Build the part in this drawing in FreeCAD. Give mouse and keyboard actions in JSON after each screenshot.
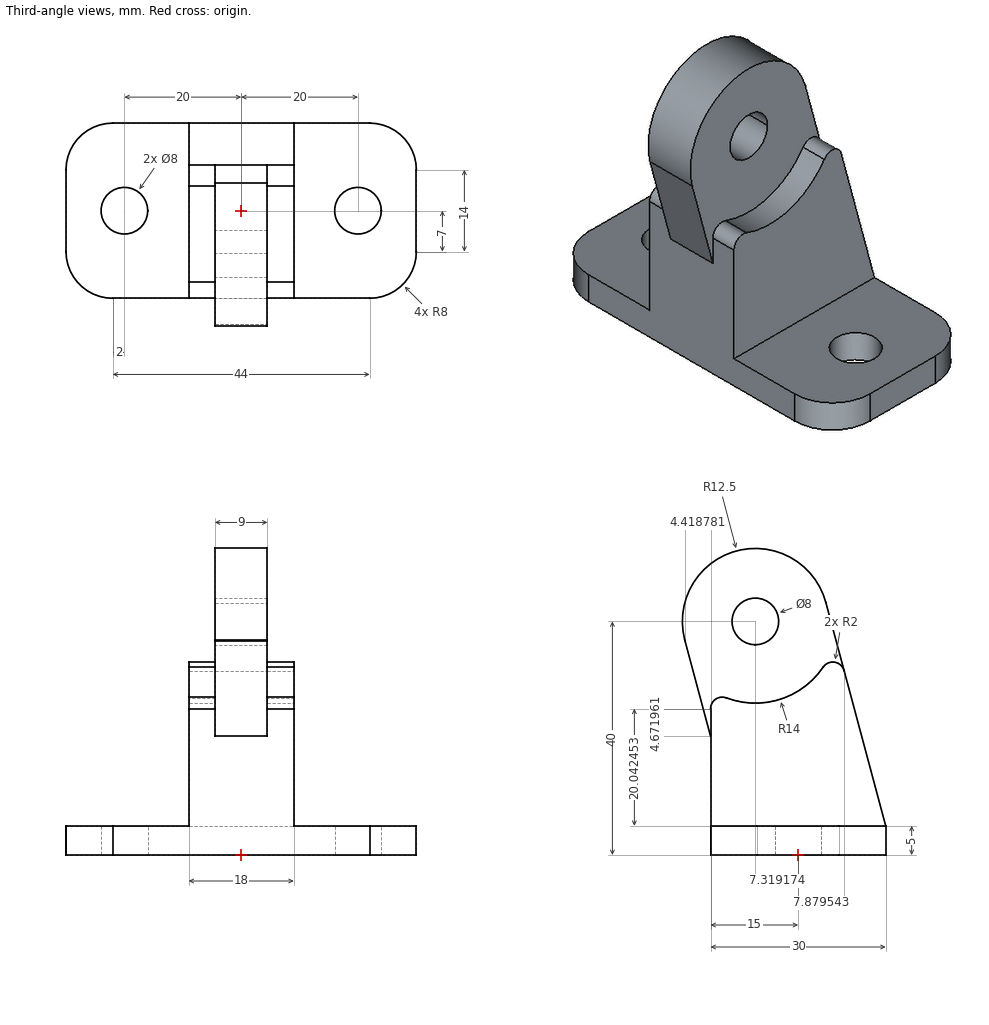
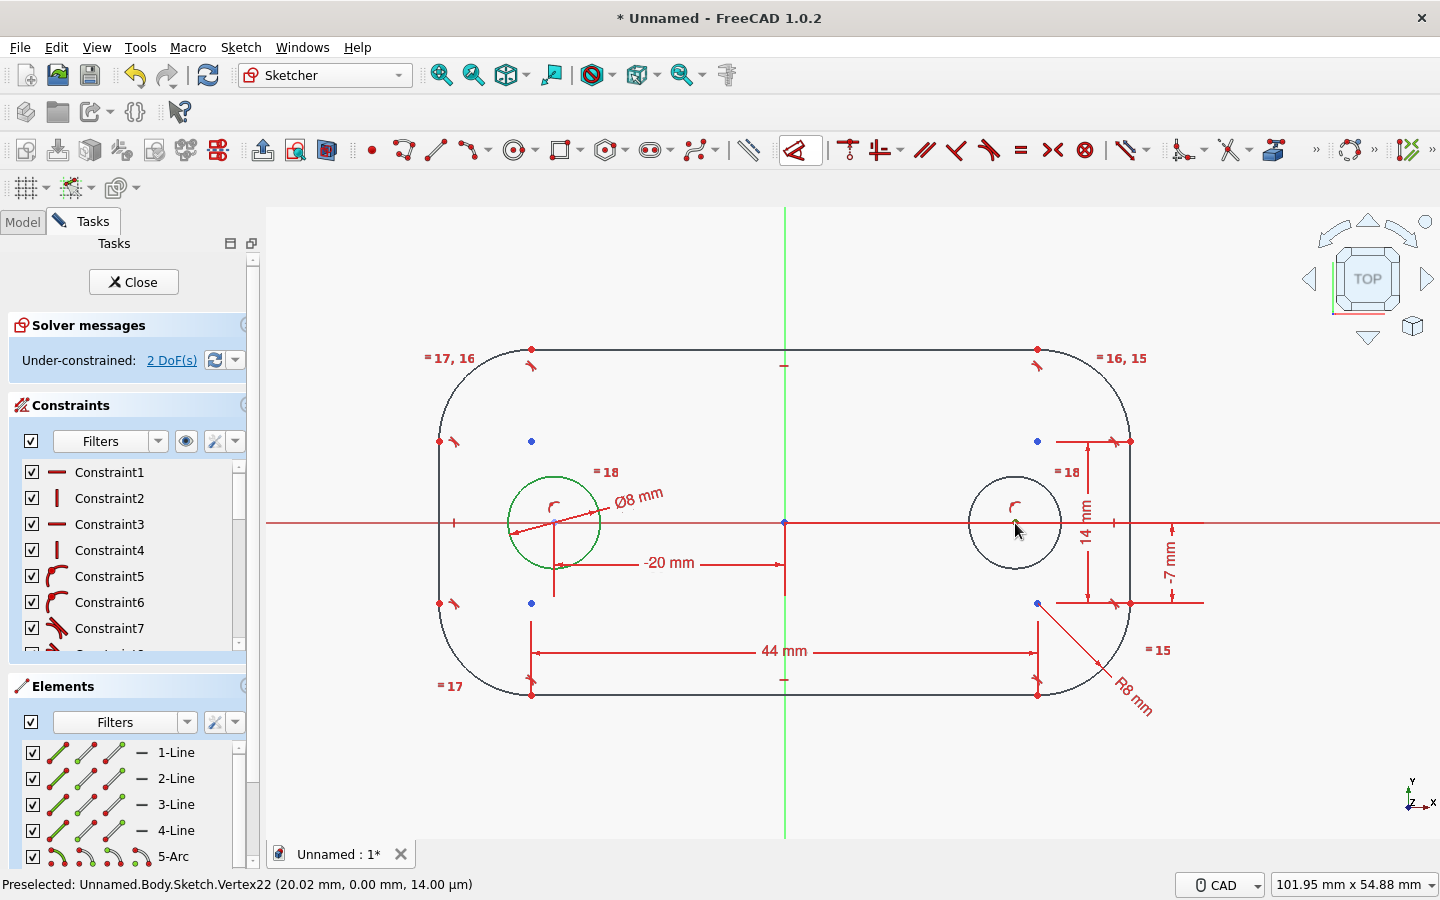
{"action": "key", "text": "l"}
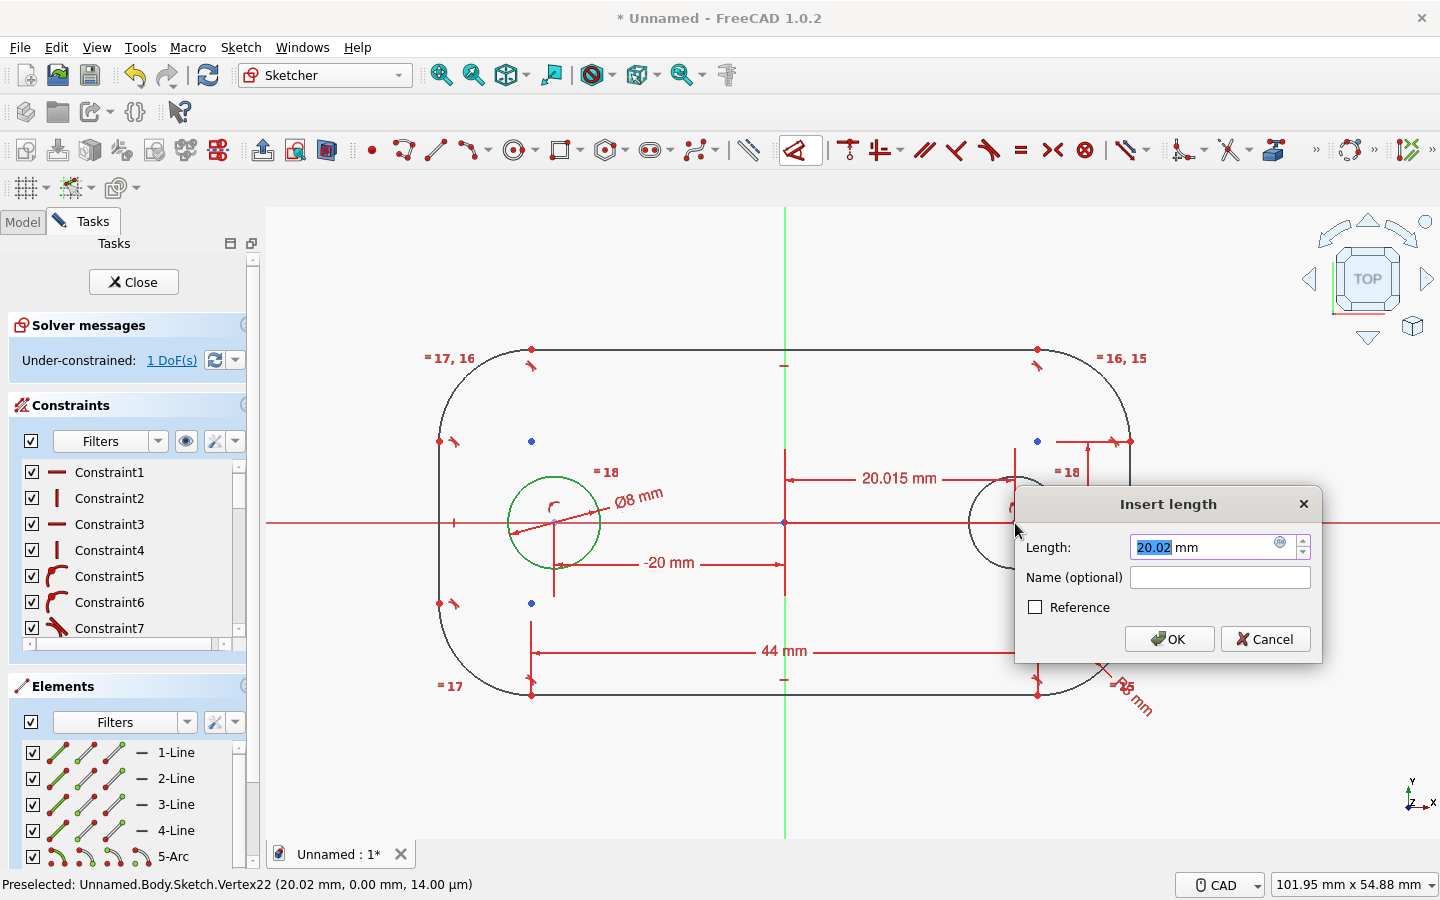
{"action": "type", "text": "20"}
{"action": "key", "text": "Return"}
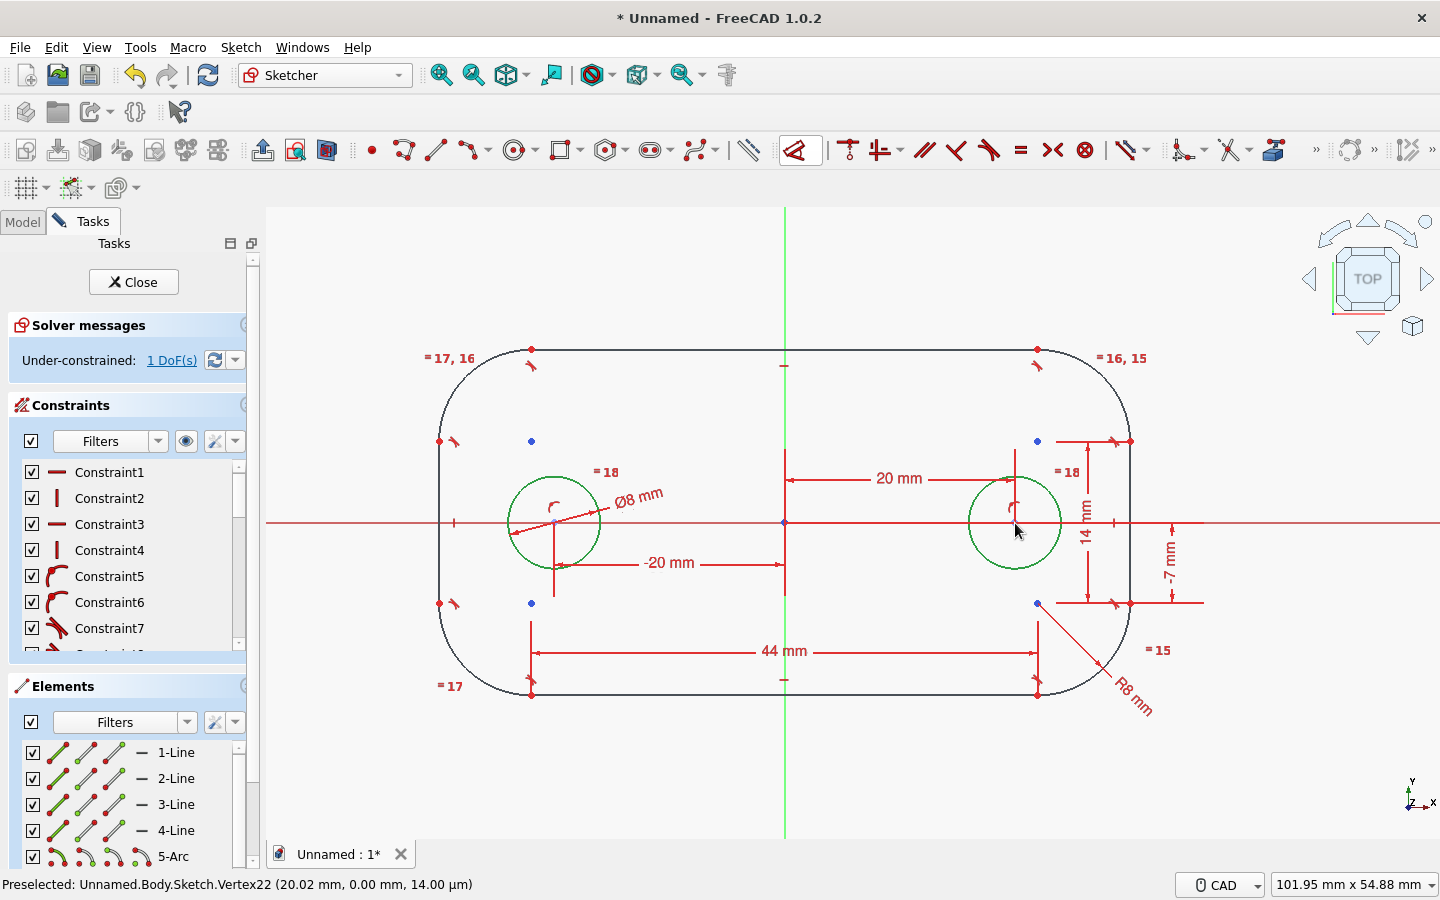
{"action": "scroll", "coordinate": [531, 695], "scroll_direction": "up", "scroll_amount": 3}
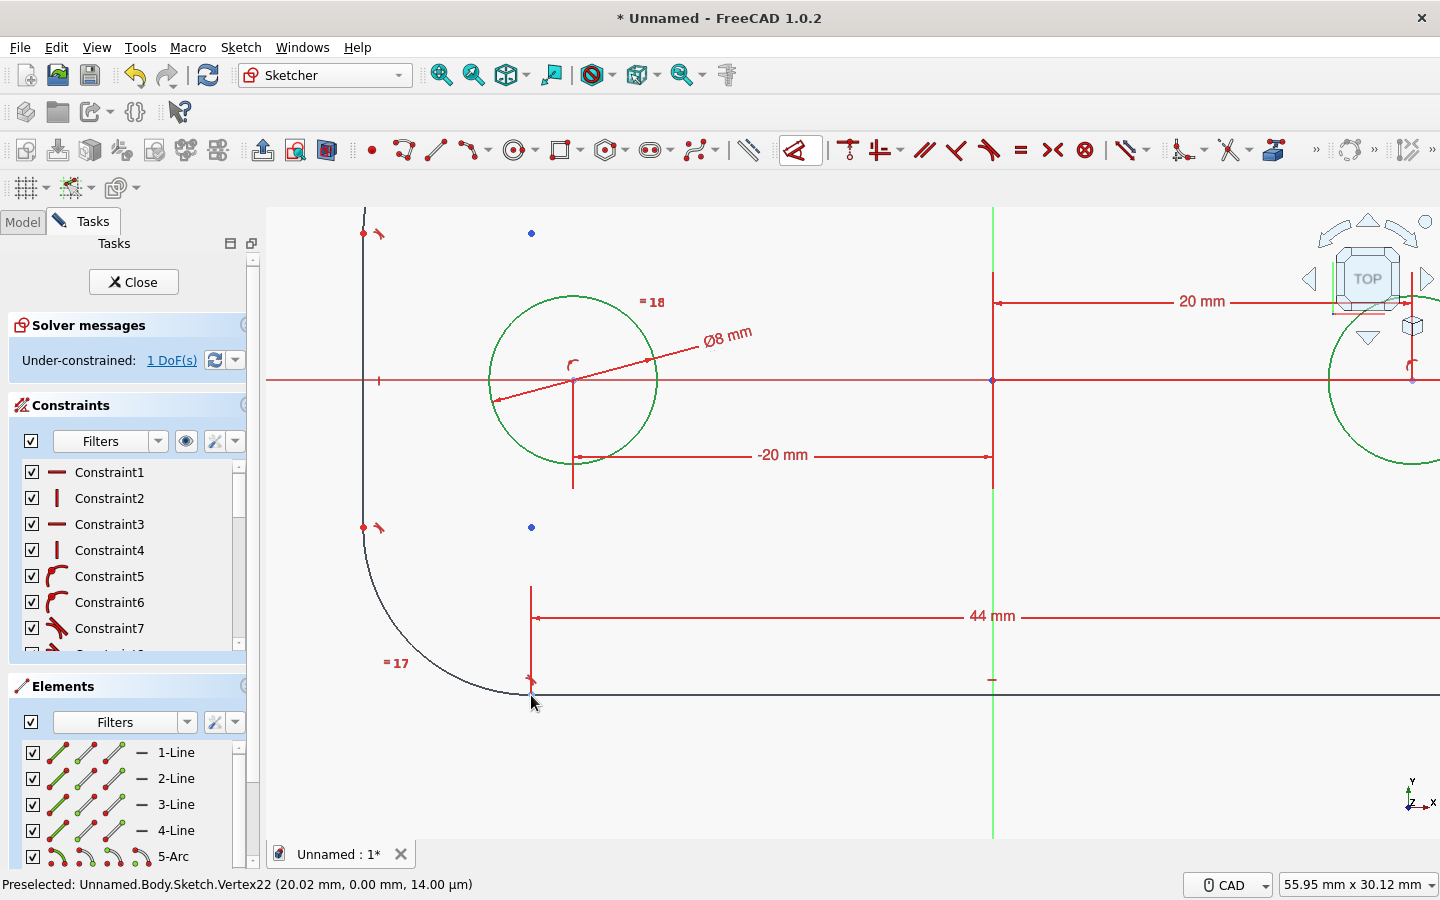
{"action": "left_click", "coordinate": [531, 695]}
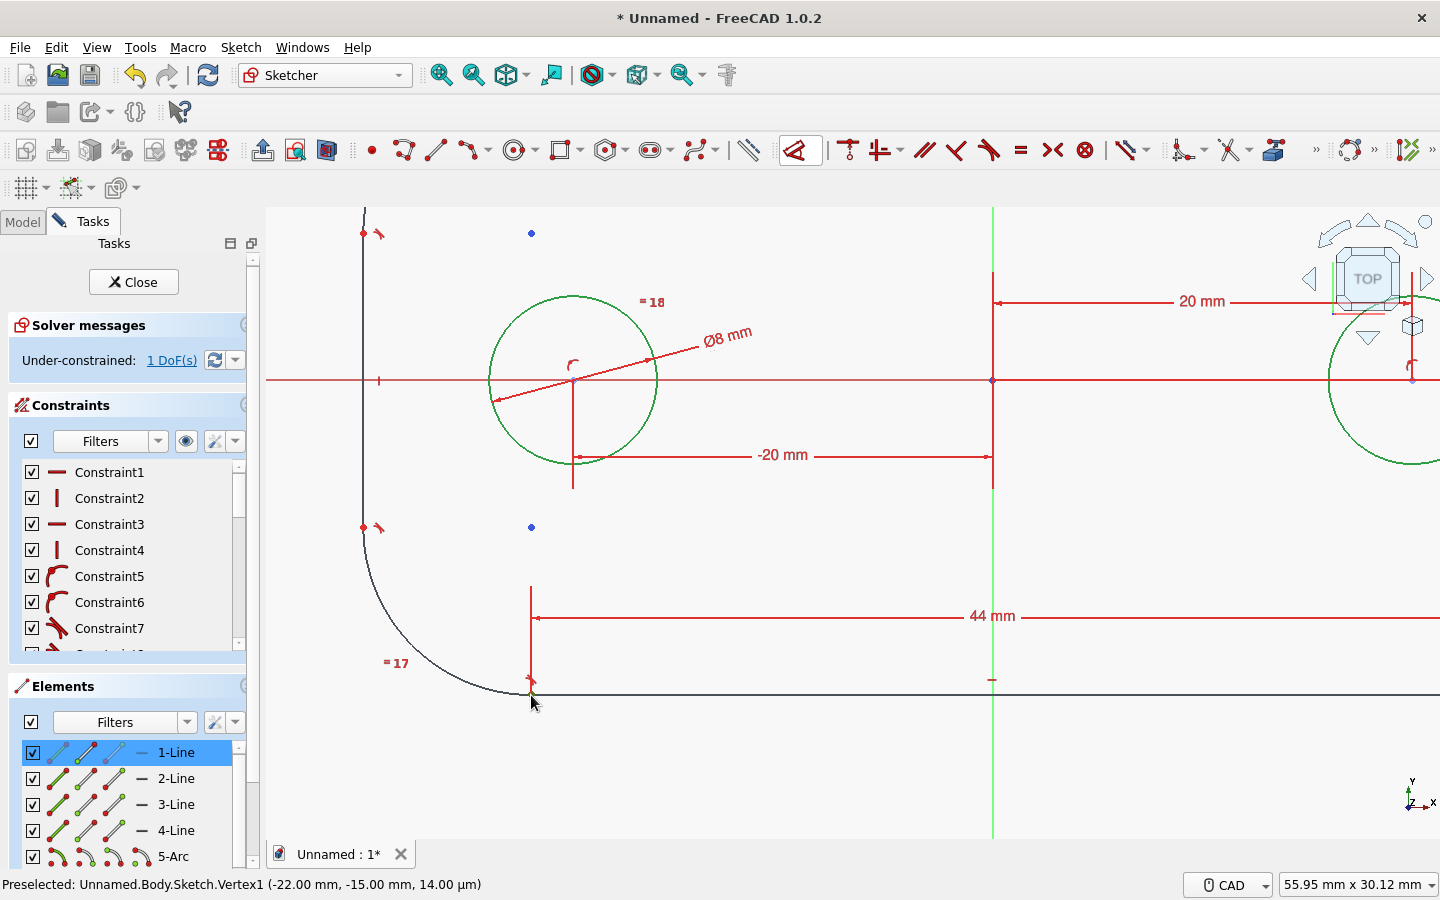
{"action": "left_click", "coordinate": [573, 380]}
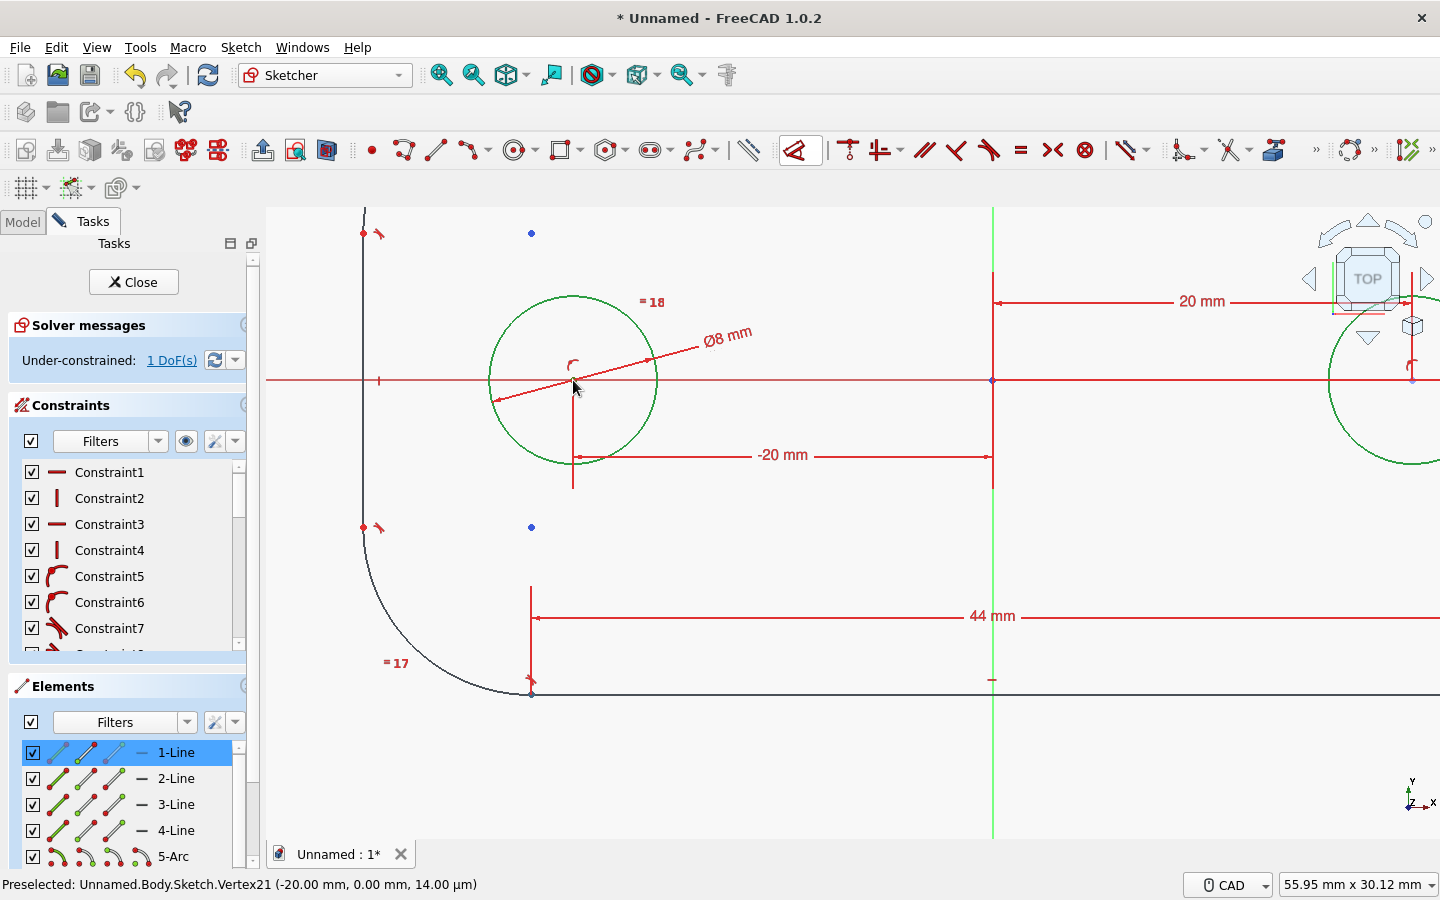
{"action": "key", "text": "l"}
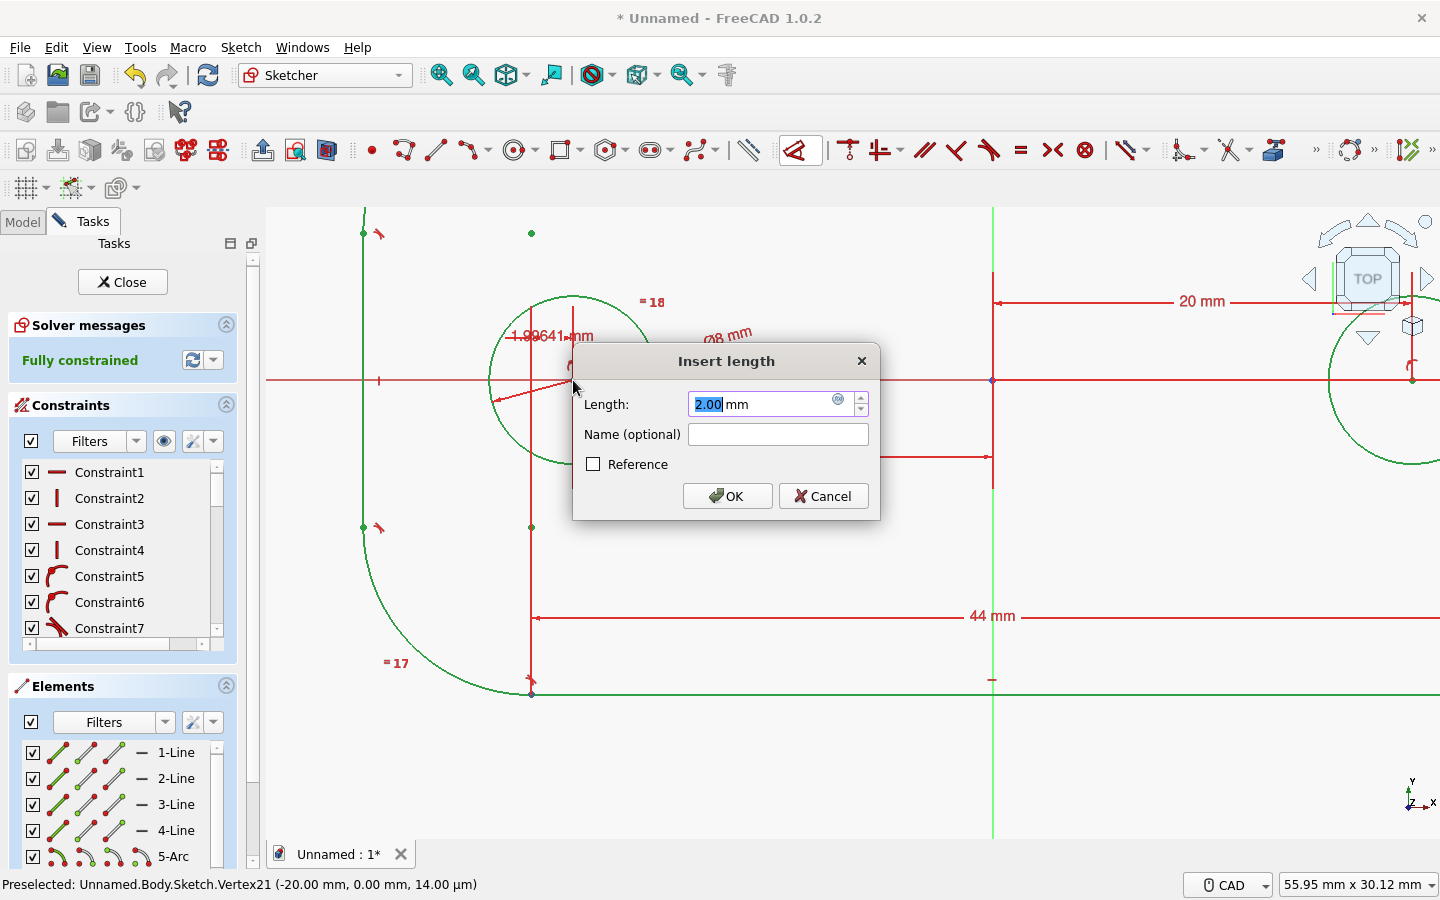
{"action": "type", "text": "2"}
{"action": "key", "text": "Return"}